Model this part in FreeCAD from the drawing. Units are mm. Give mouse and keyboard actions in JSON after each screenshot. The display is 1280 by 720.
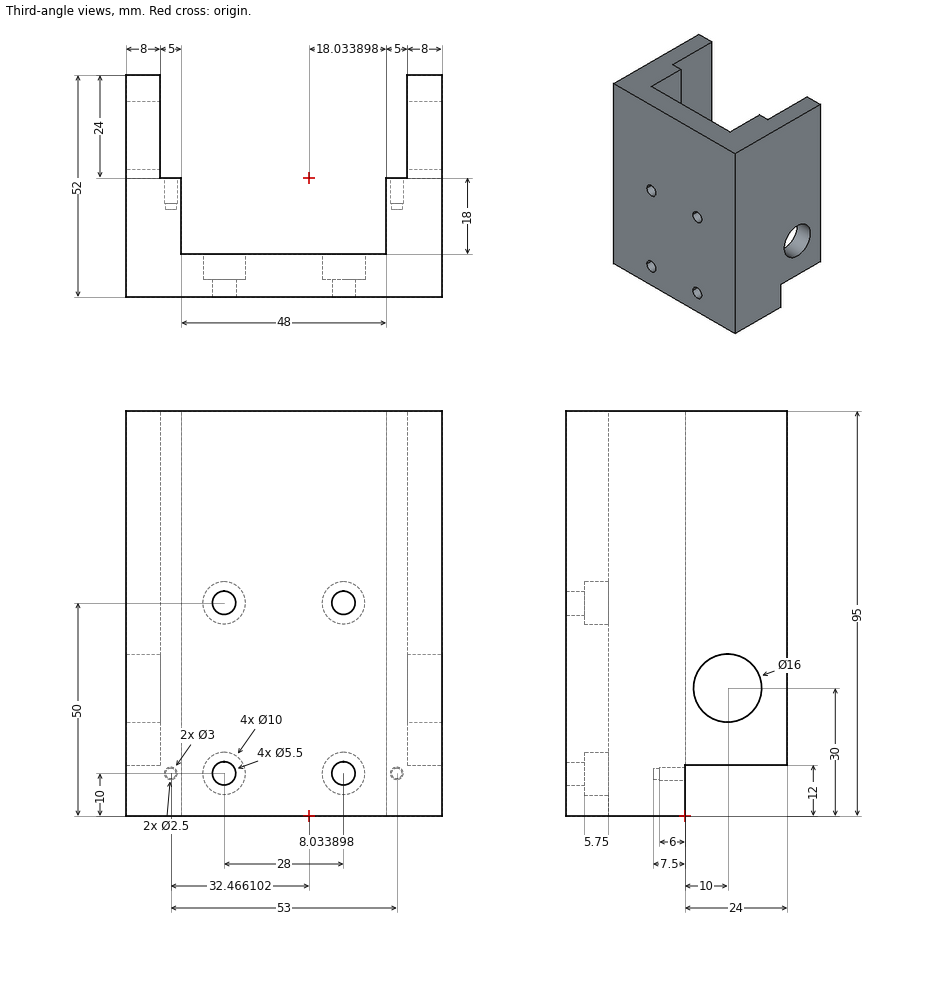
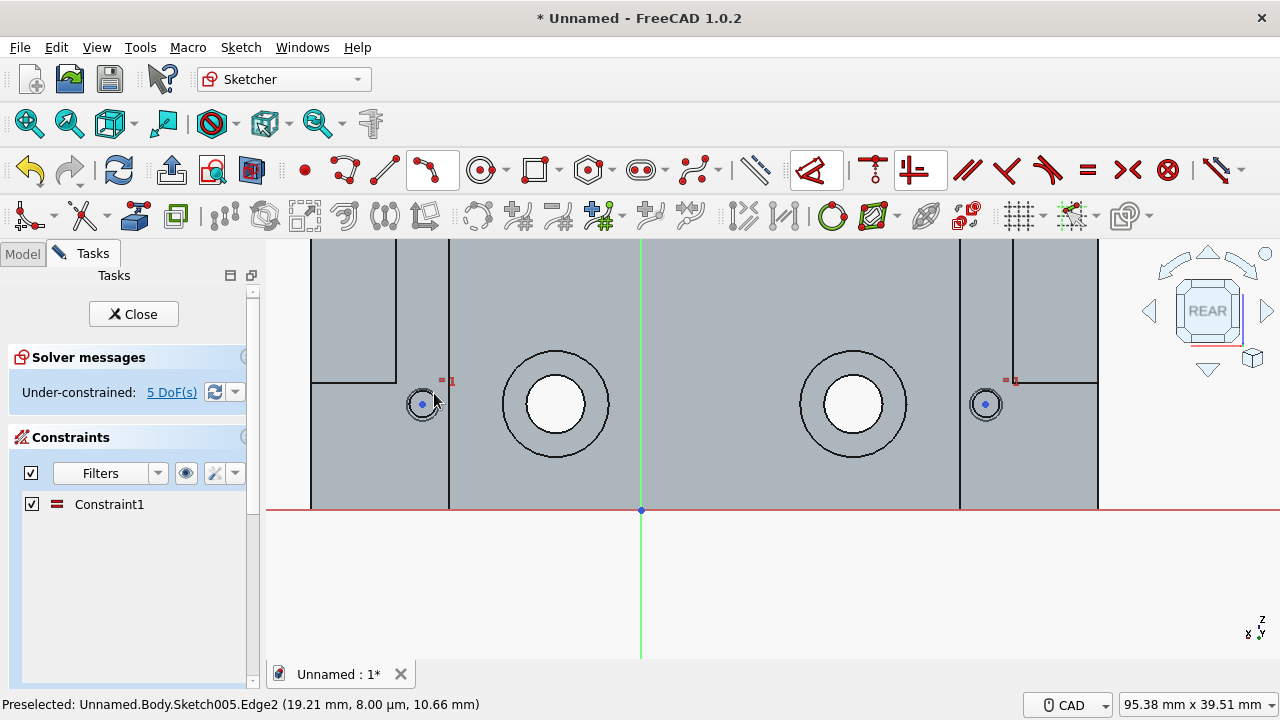
{"action": "left_click", "coordinate": [986, 405]}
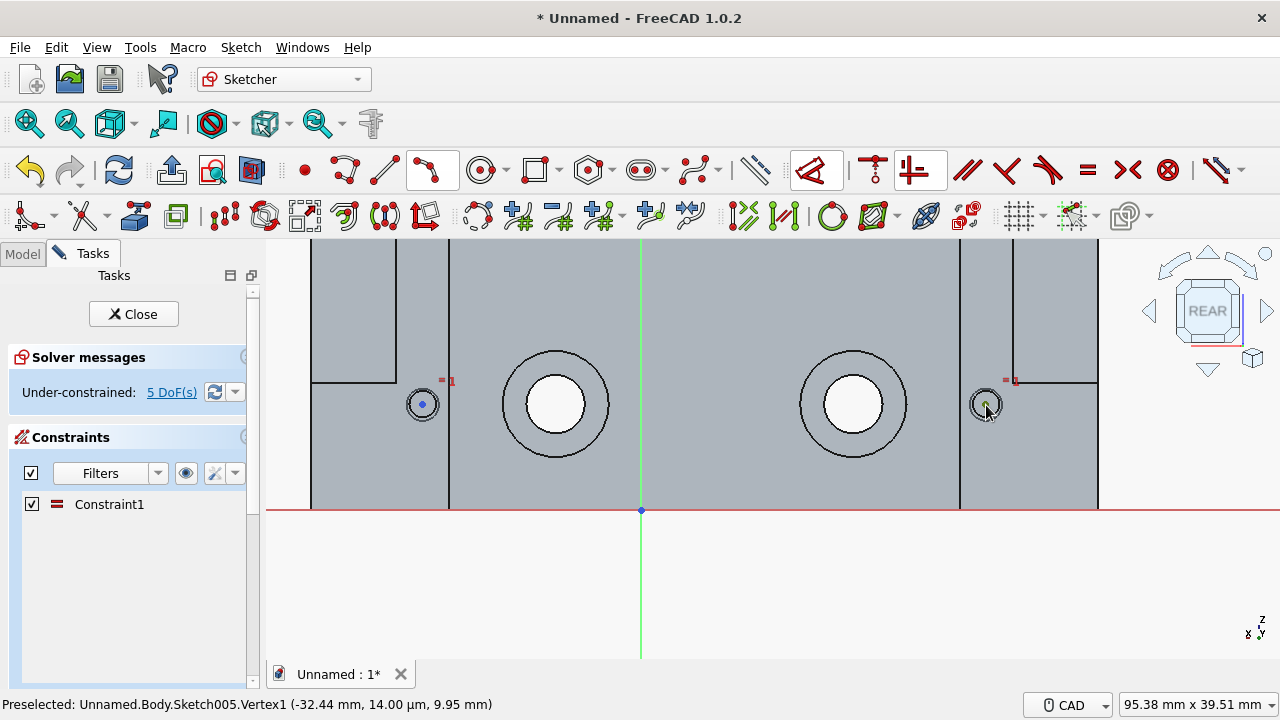
{"action": "left_click", "coordinate": [423, 405]}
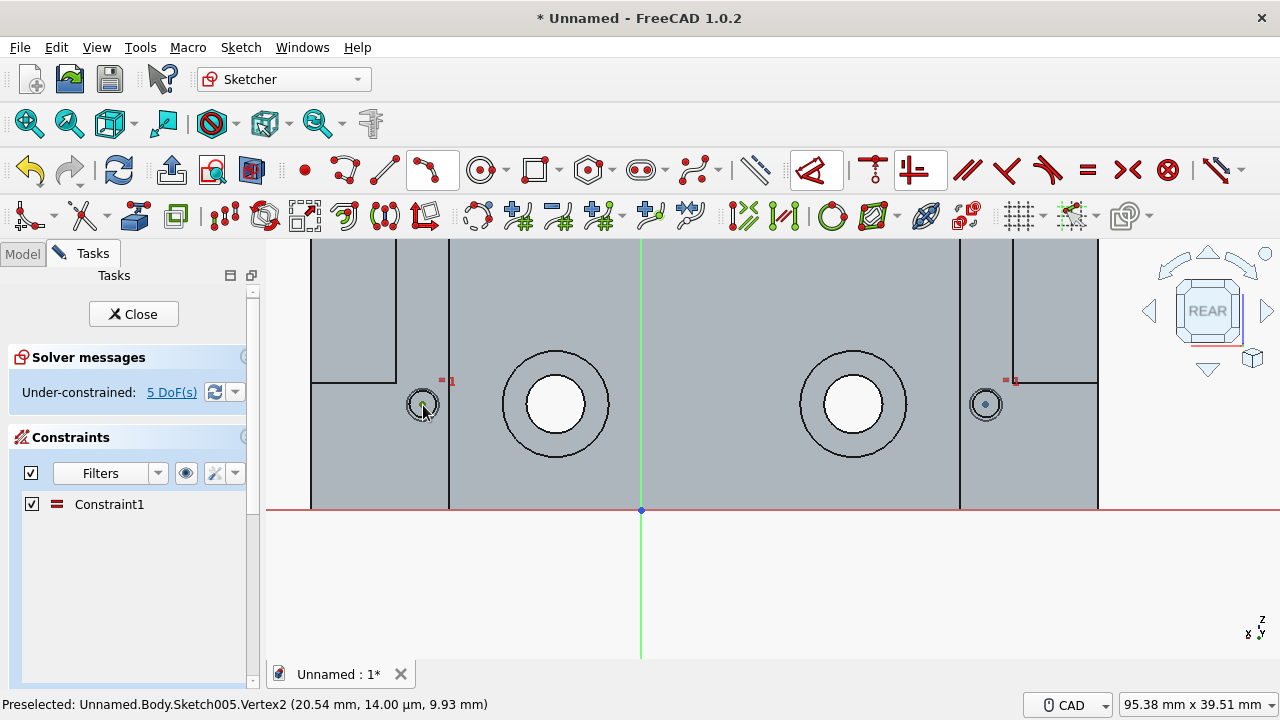
{"action": "key", "text": "h"}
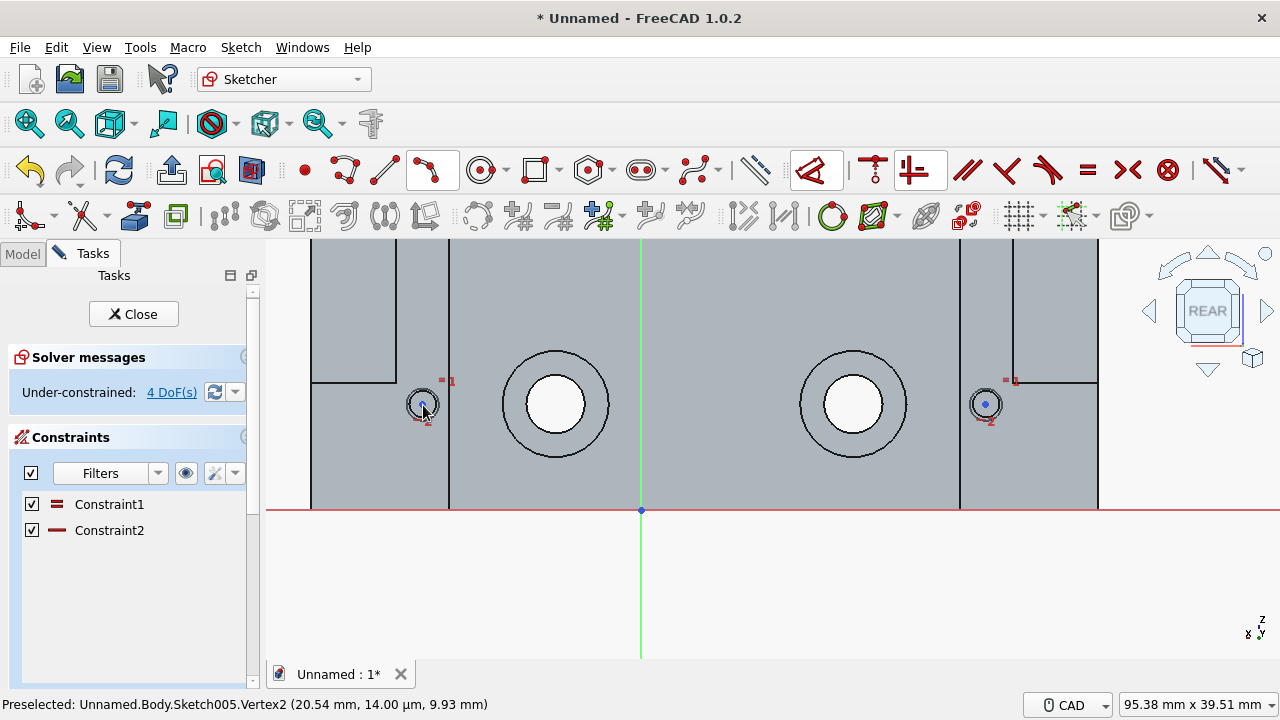
{"action": "scroll", "coordinate": [997, 393], "scroll_direction": "up", "scroll_amount": 2}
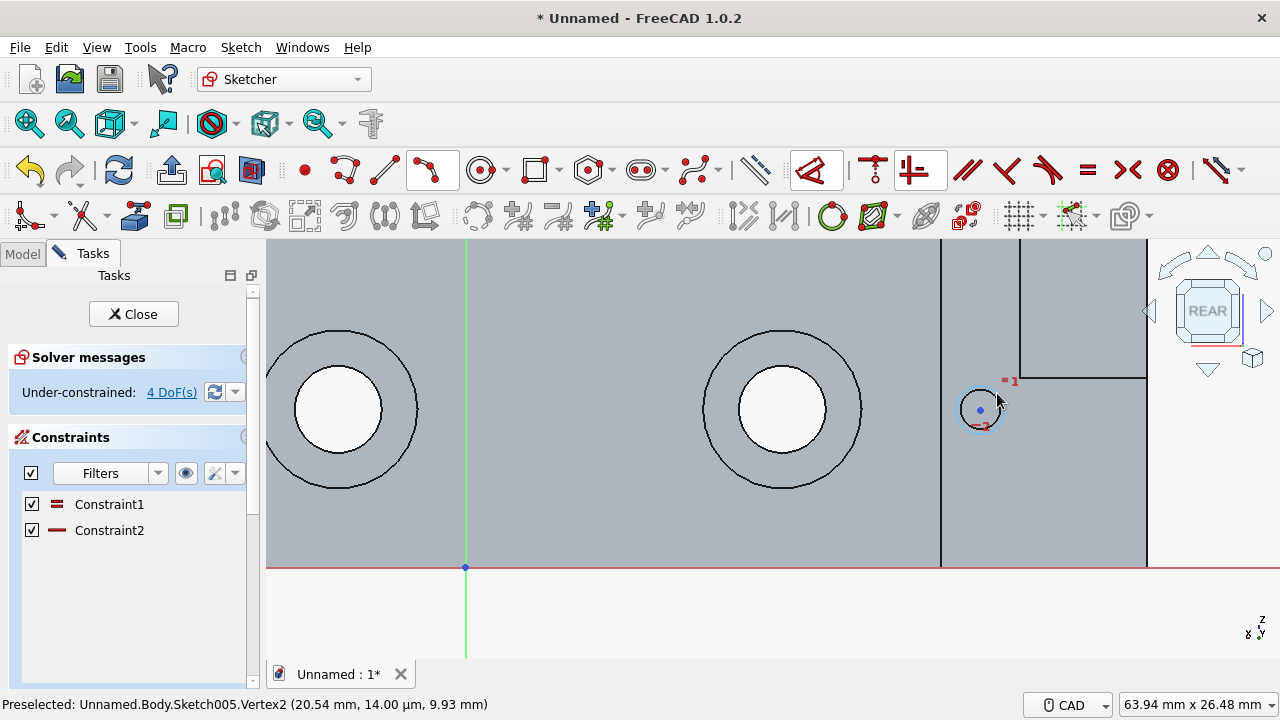
{"action": "left_click", "coordinate": [997, 393]}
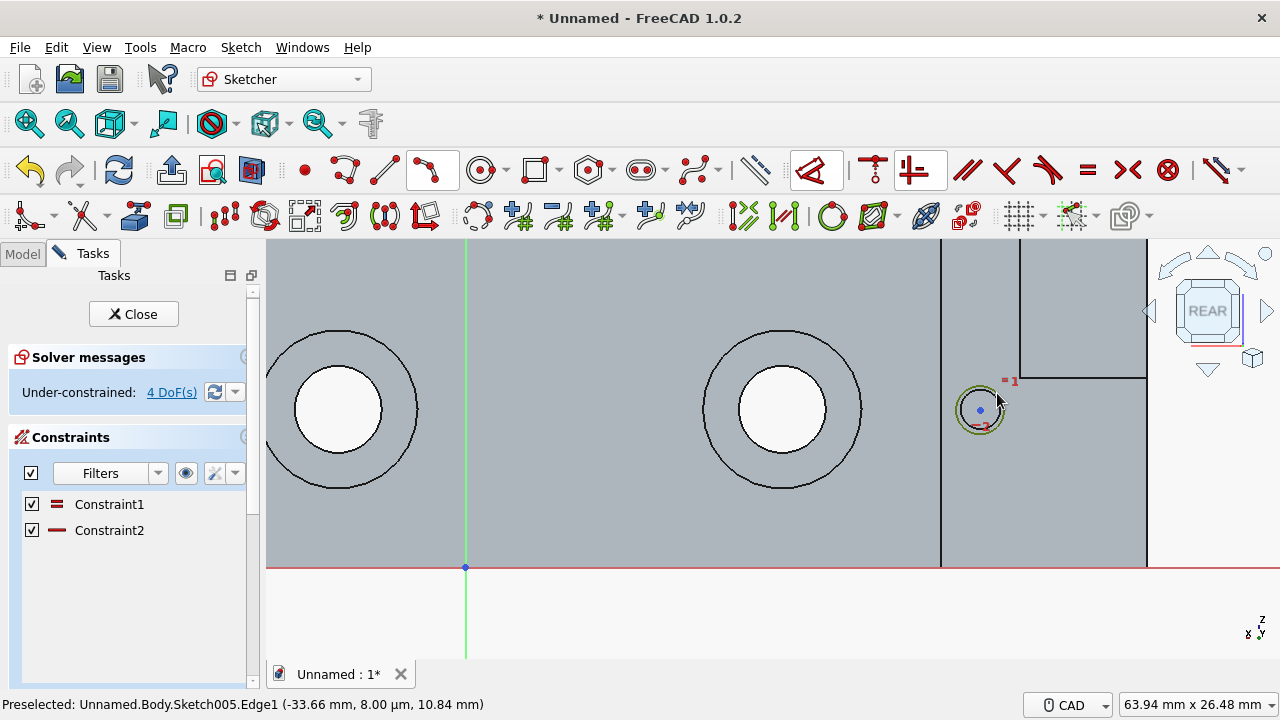
{"action": "key", "text": "k o"}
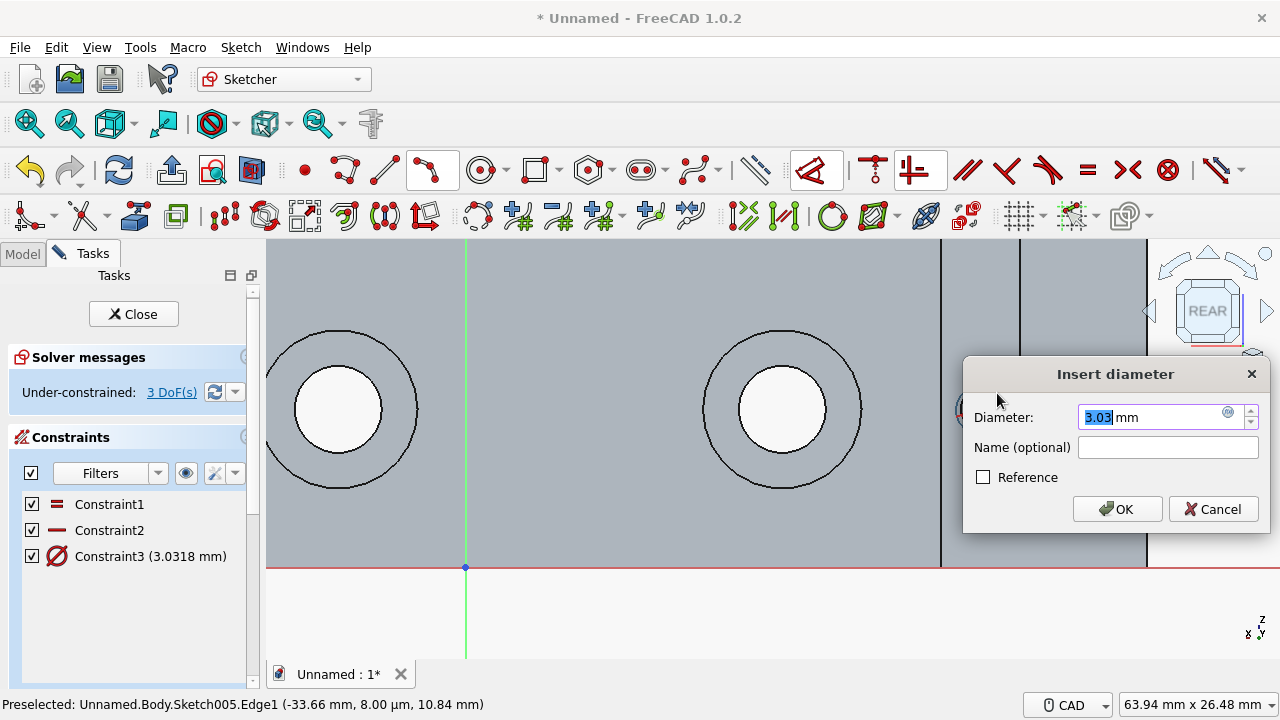
{"action": "type", "text": "3"}
{"action": "key", "text": "Return"}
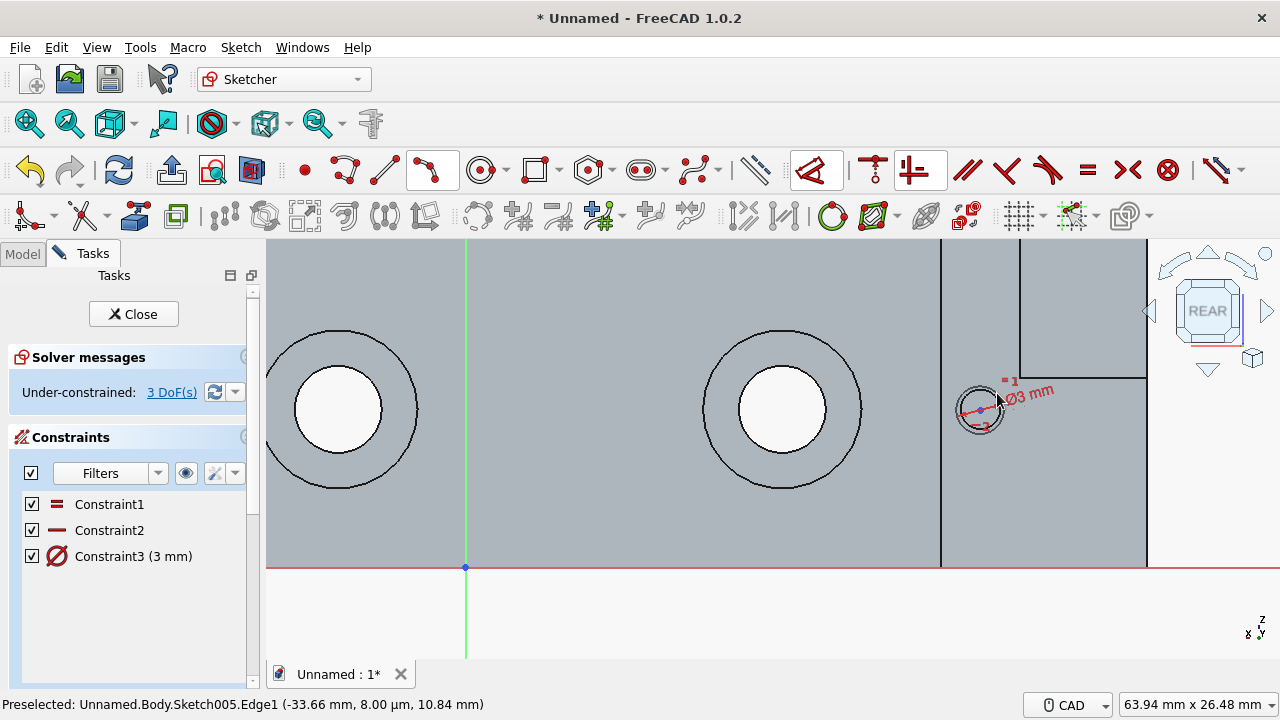
{"action": "left_click", "coordinate": [980, 410]}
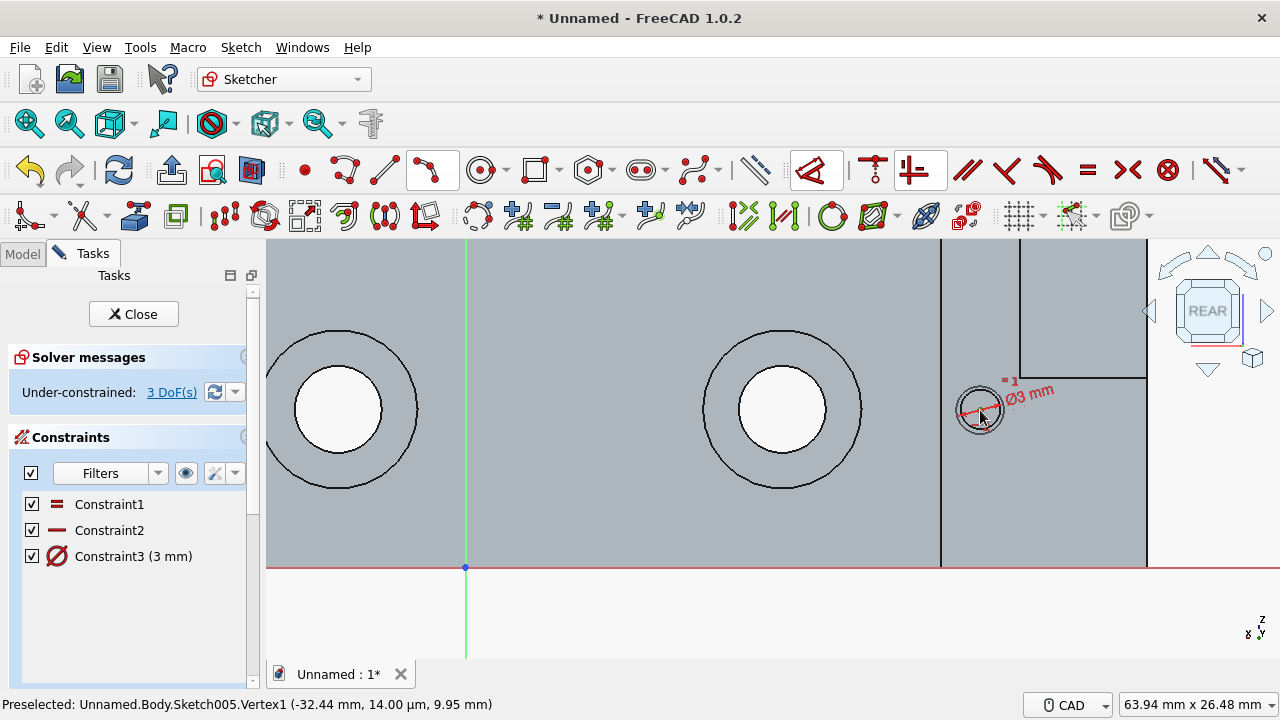
{"action": "key", "text": "i"}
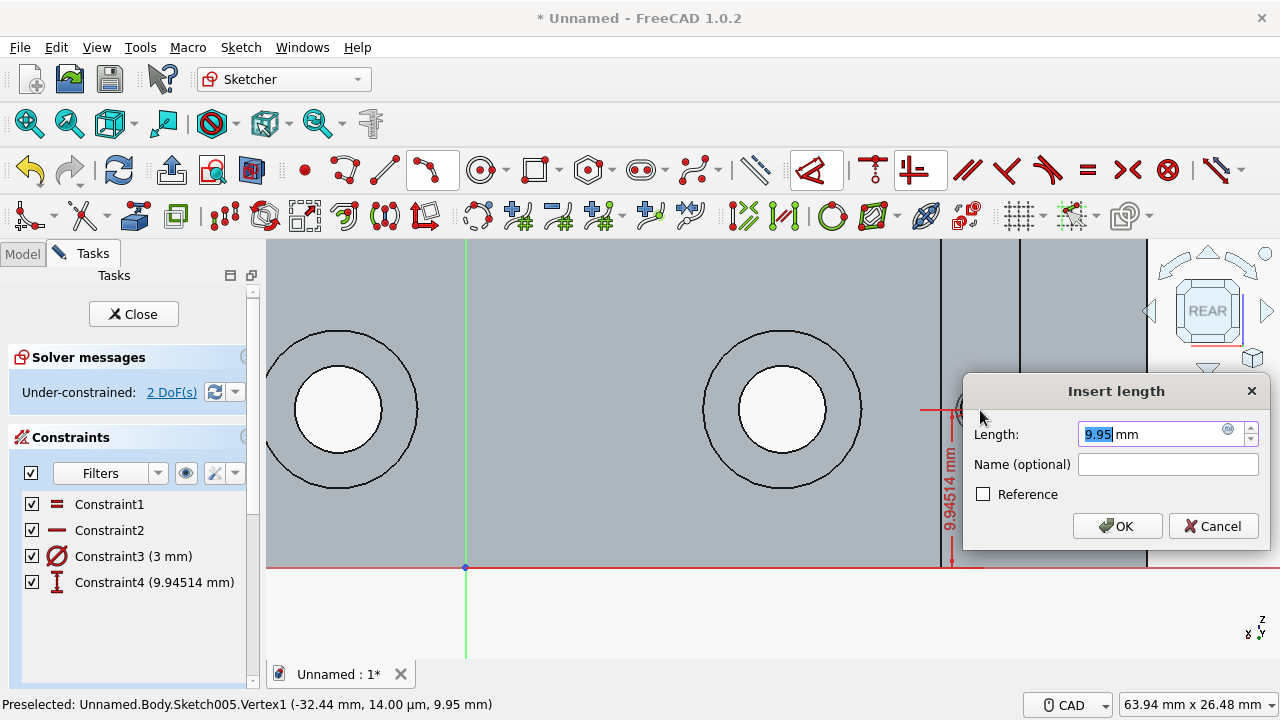
{"action": "type", "text": "10"}
{"action": "key", "text": "Return"}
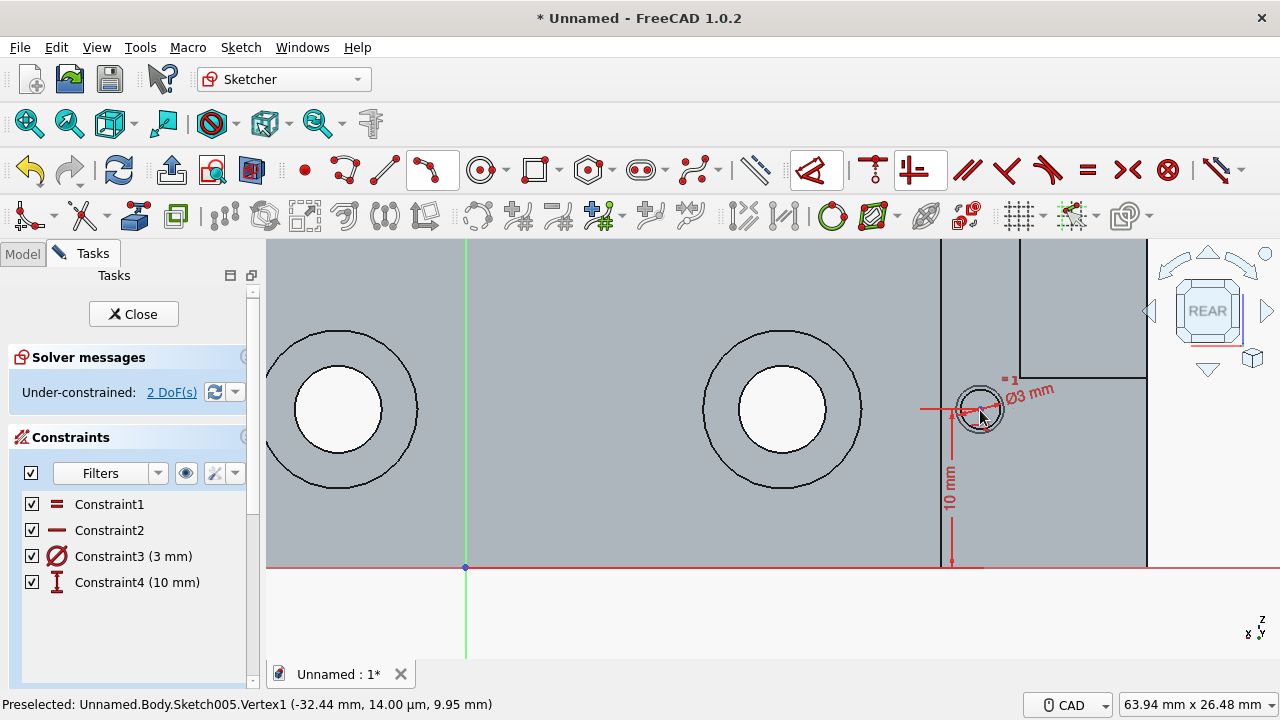
{"action": "left_click", "coordinate": [980, 409]}